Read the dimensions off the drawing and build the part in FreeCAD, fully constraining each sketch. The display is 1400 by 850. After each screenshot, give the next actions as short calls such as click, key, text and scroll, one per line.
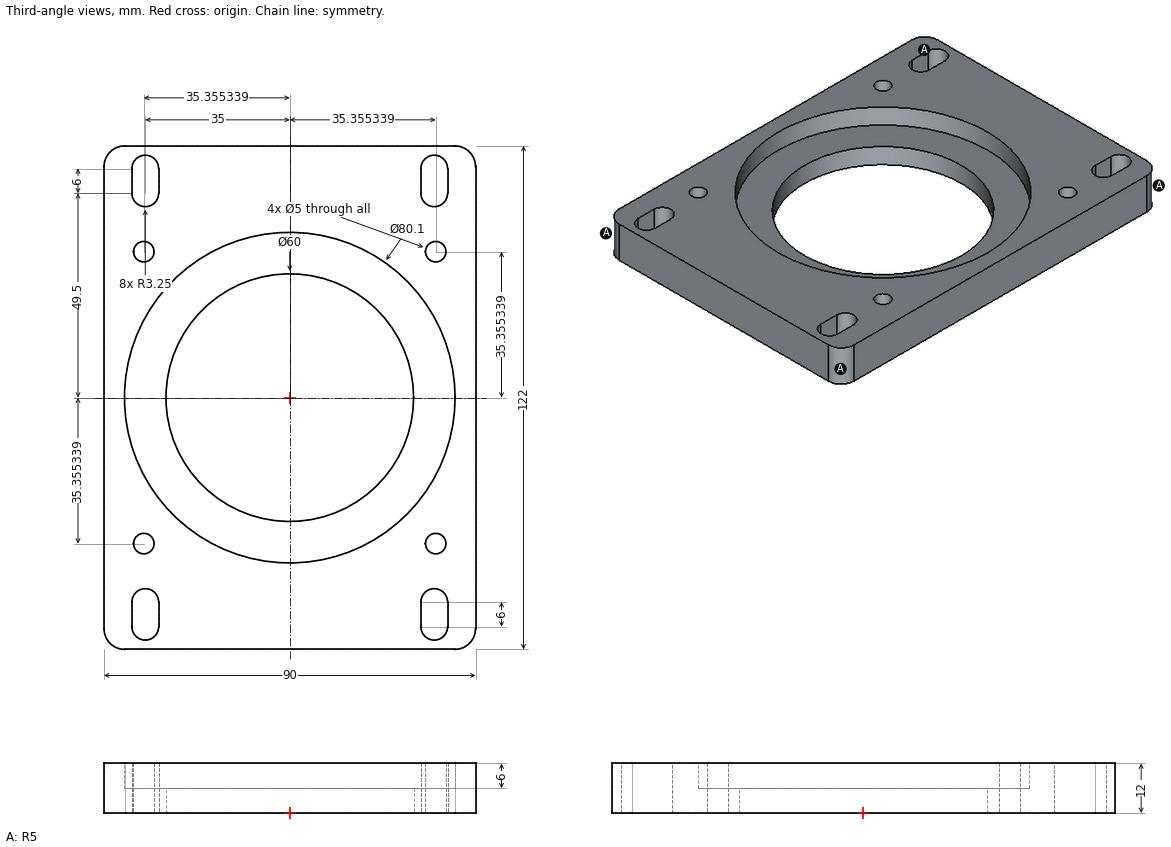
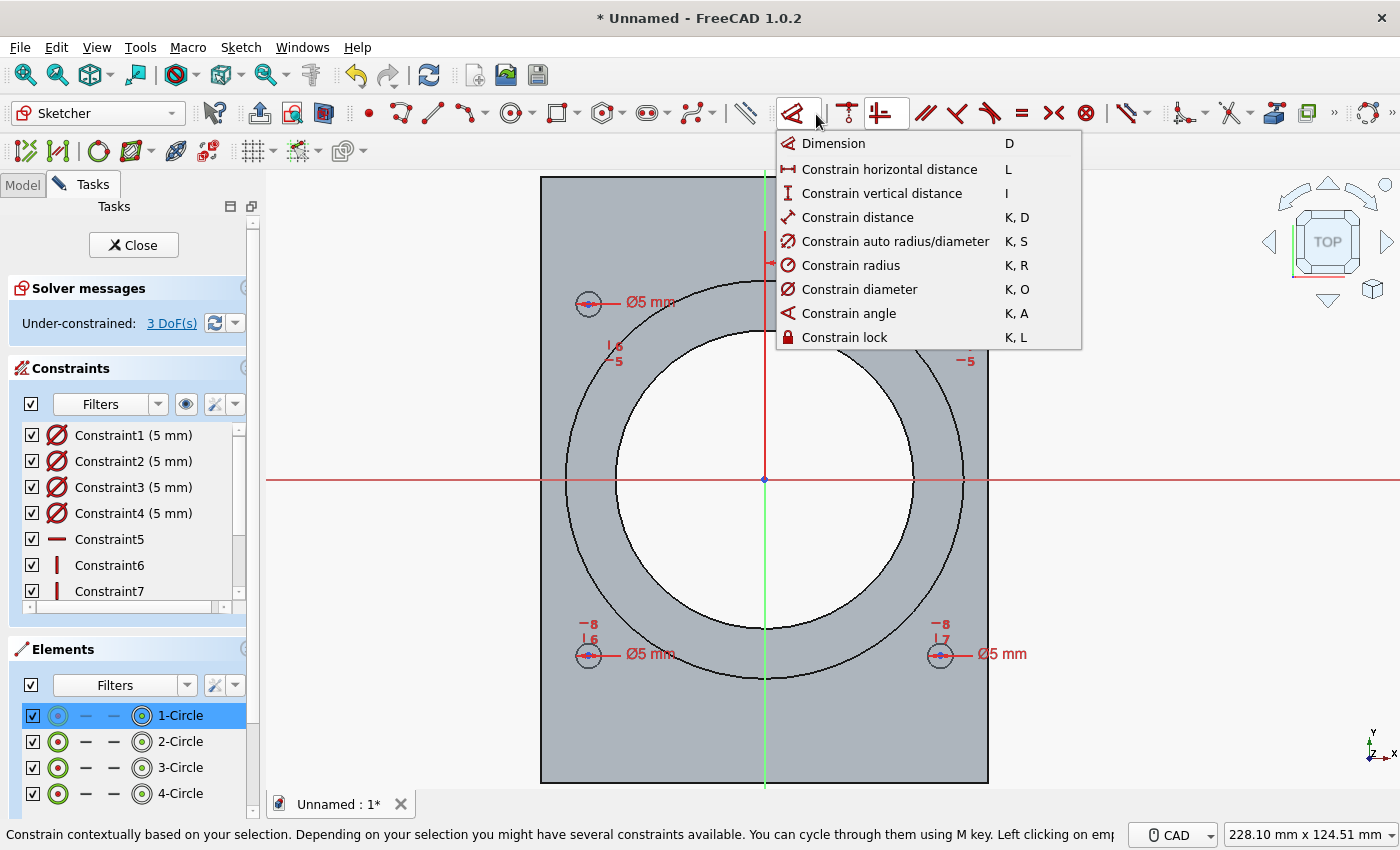
click(929, 193)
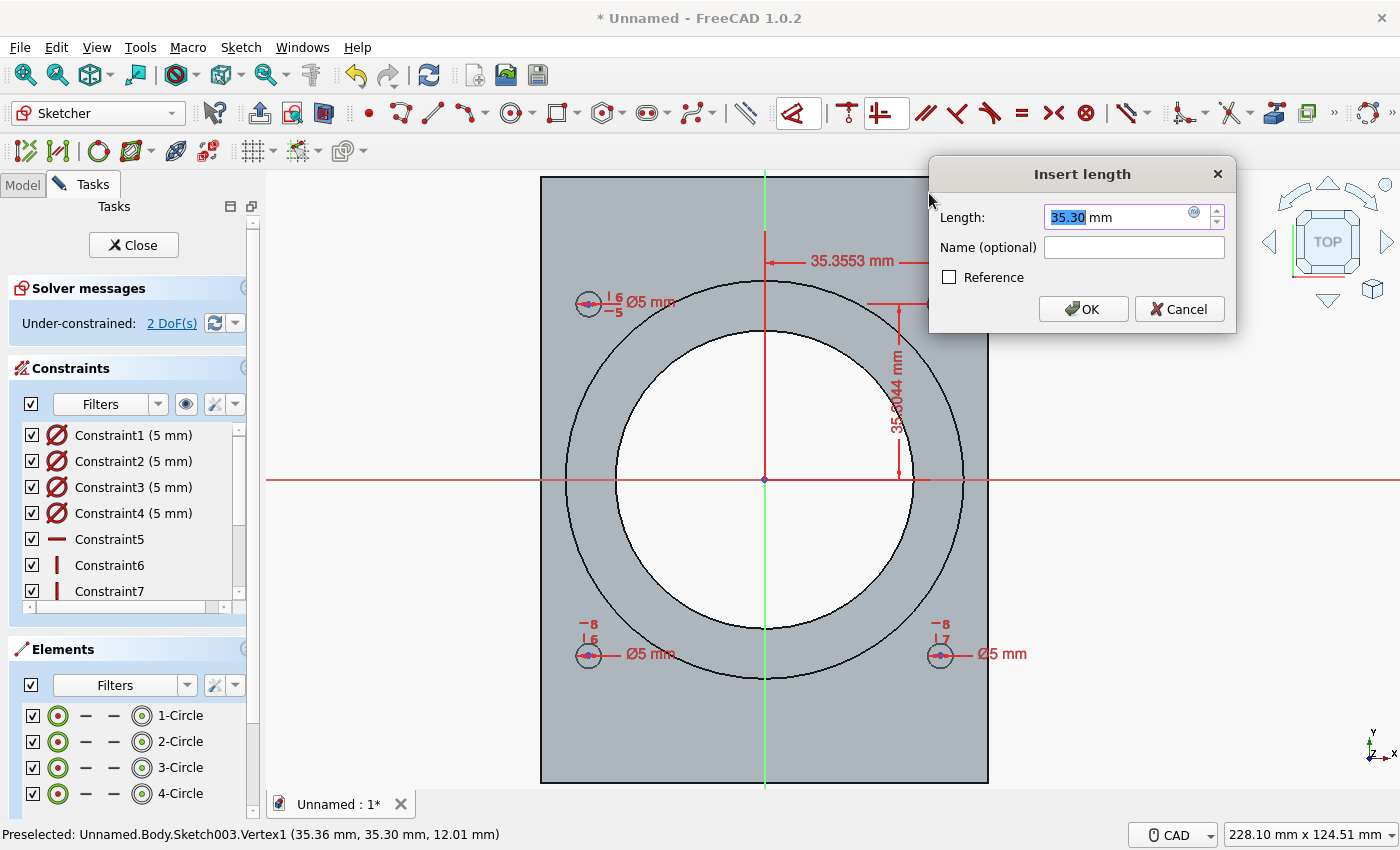
text(35.355339)
key(Return)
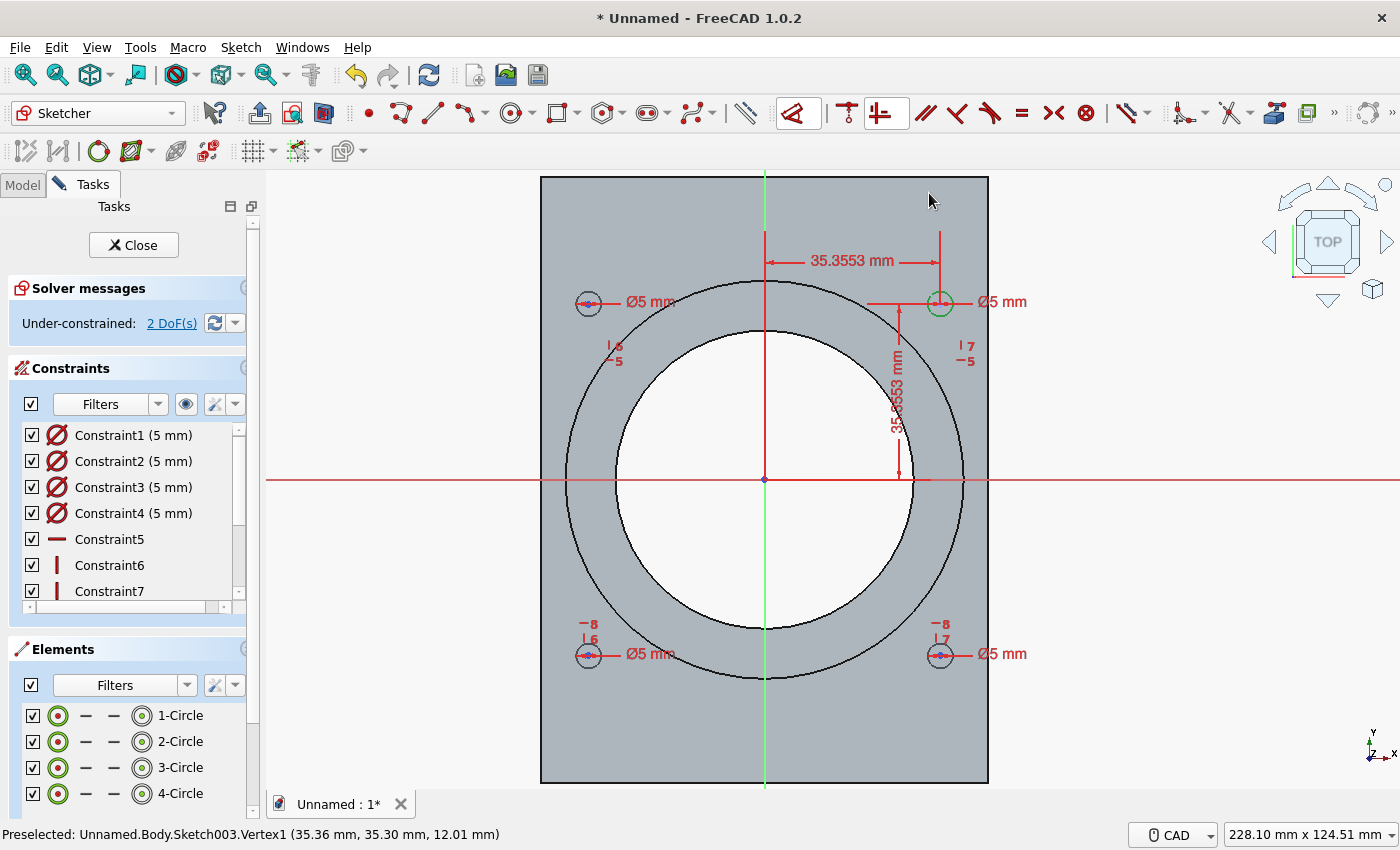
click(589, 304)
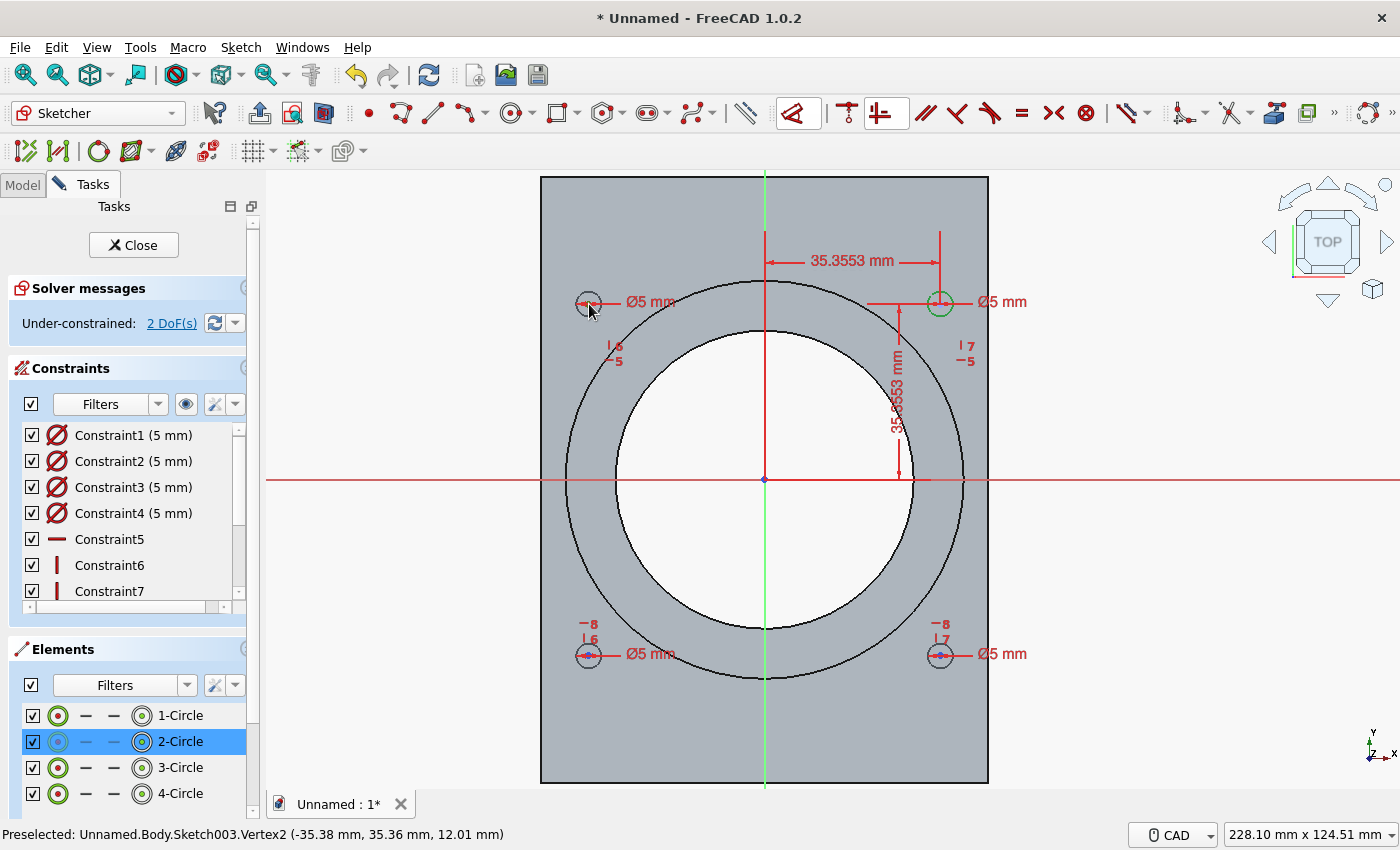
click(816, 114)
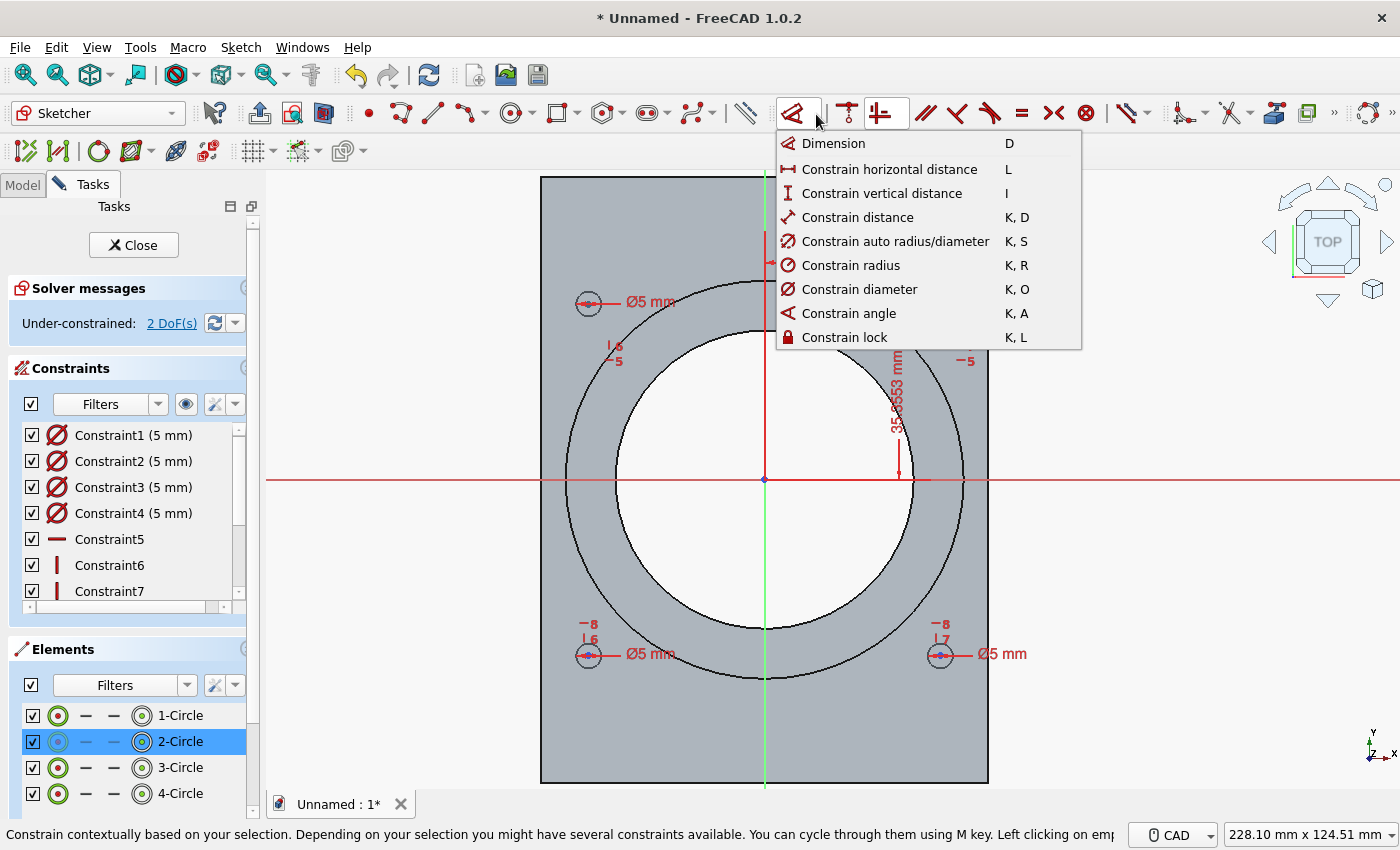
click(929, 169)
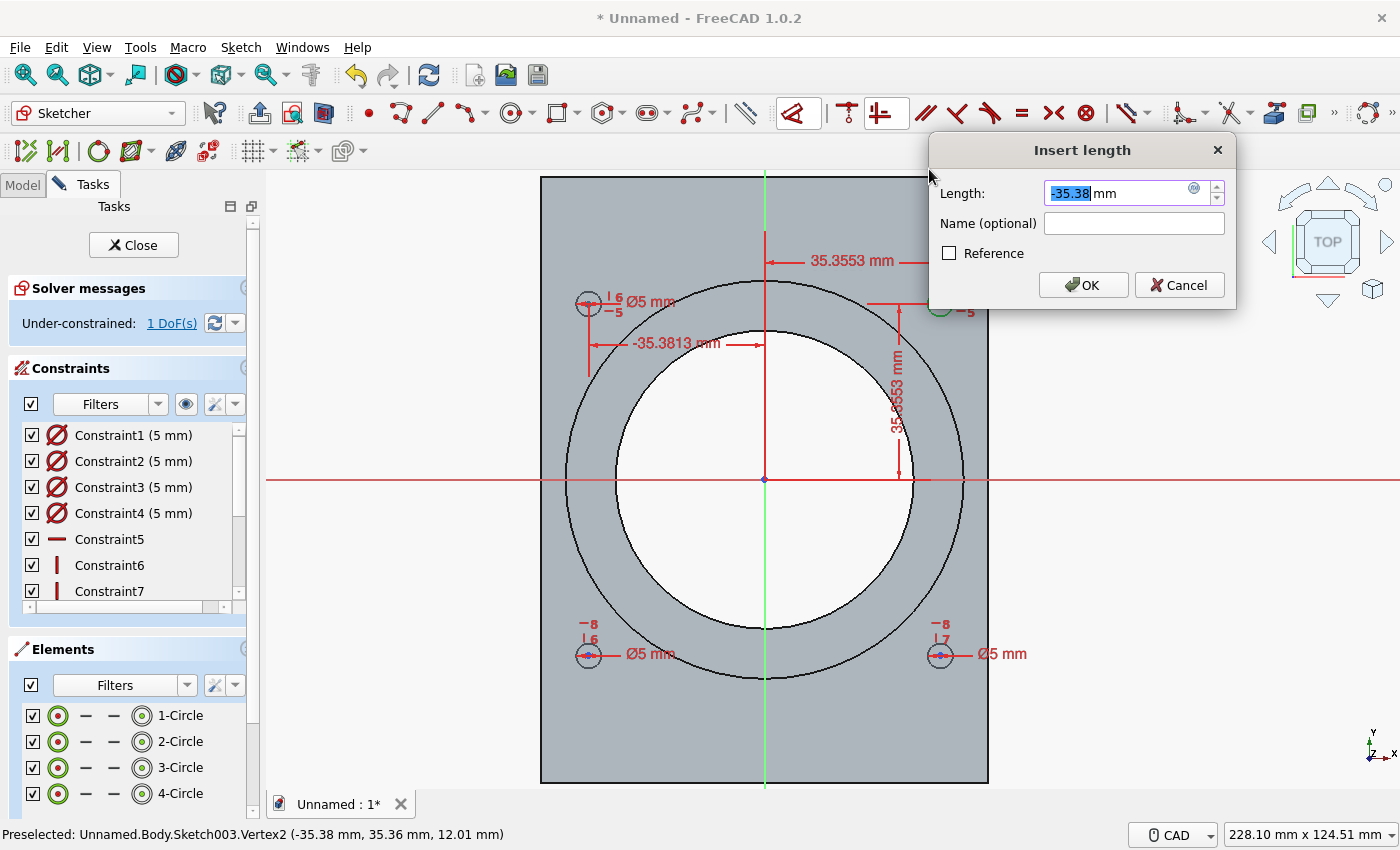
text(-35.355339)
key(Return)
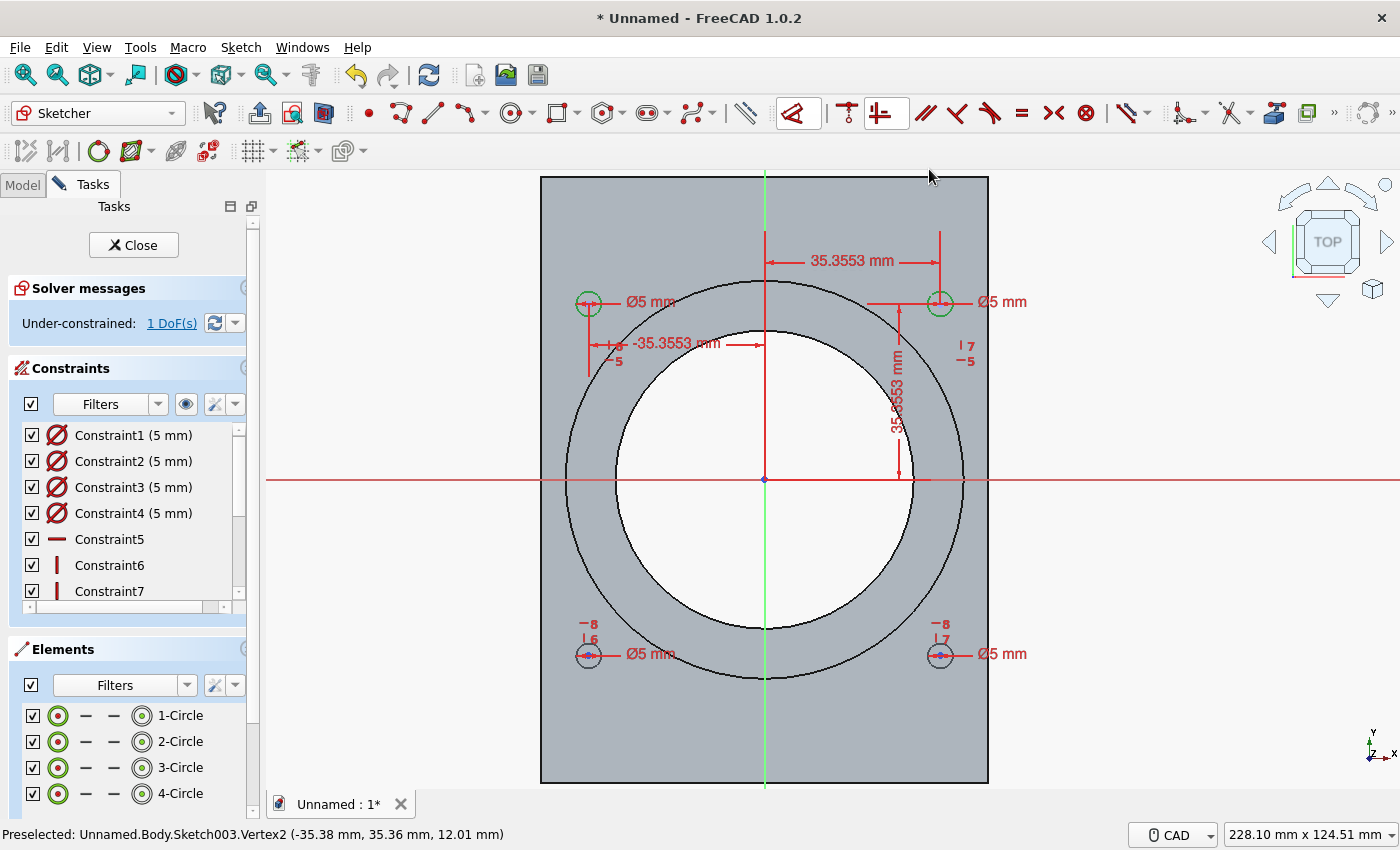
click(589, 656)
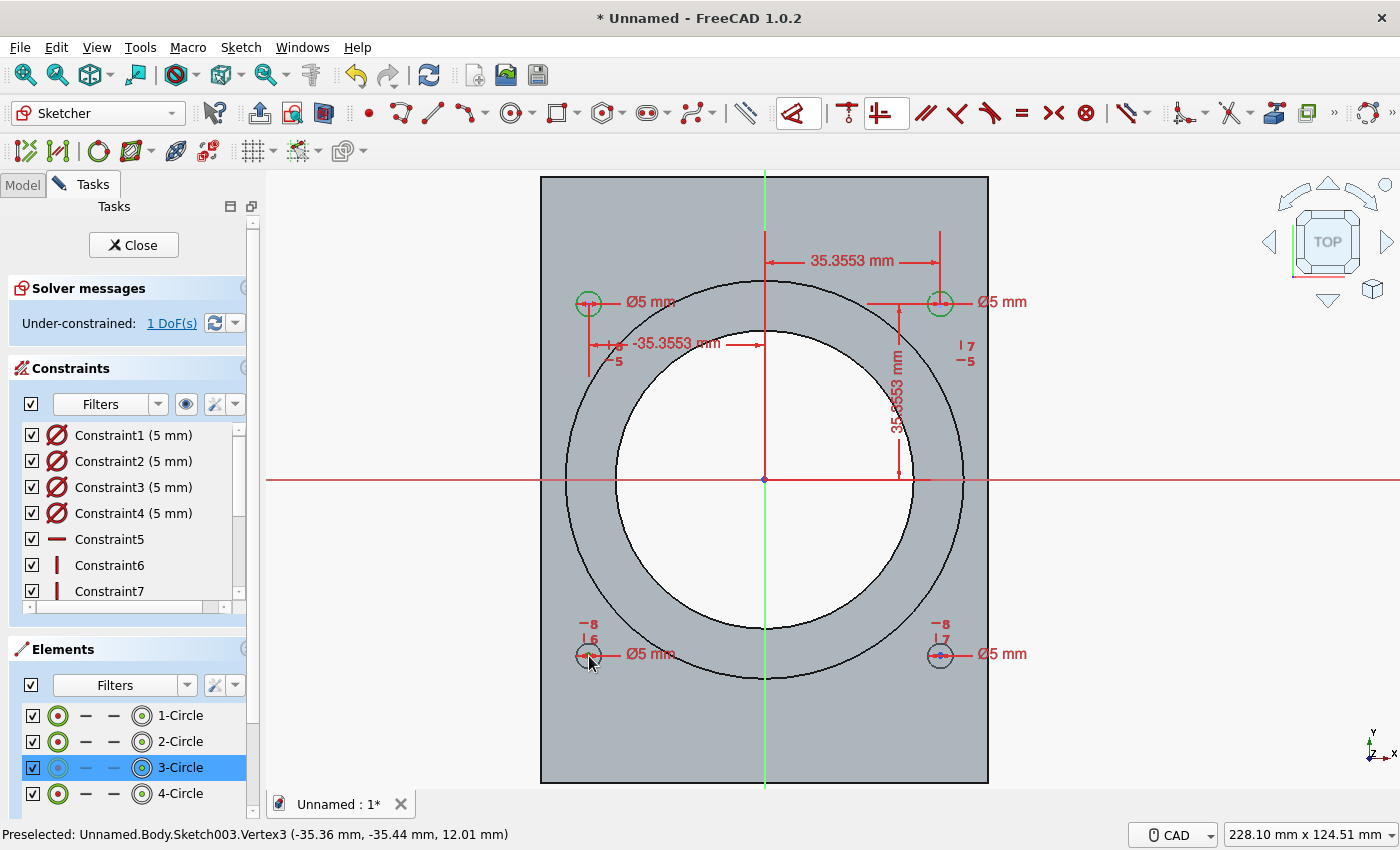
click(816, 114)